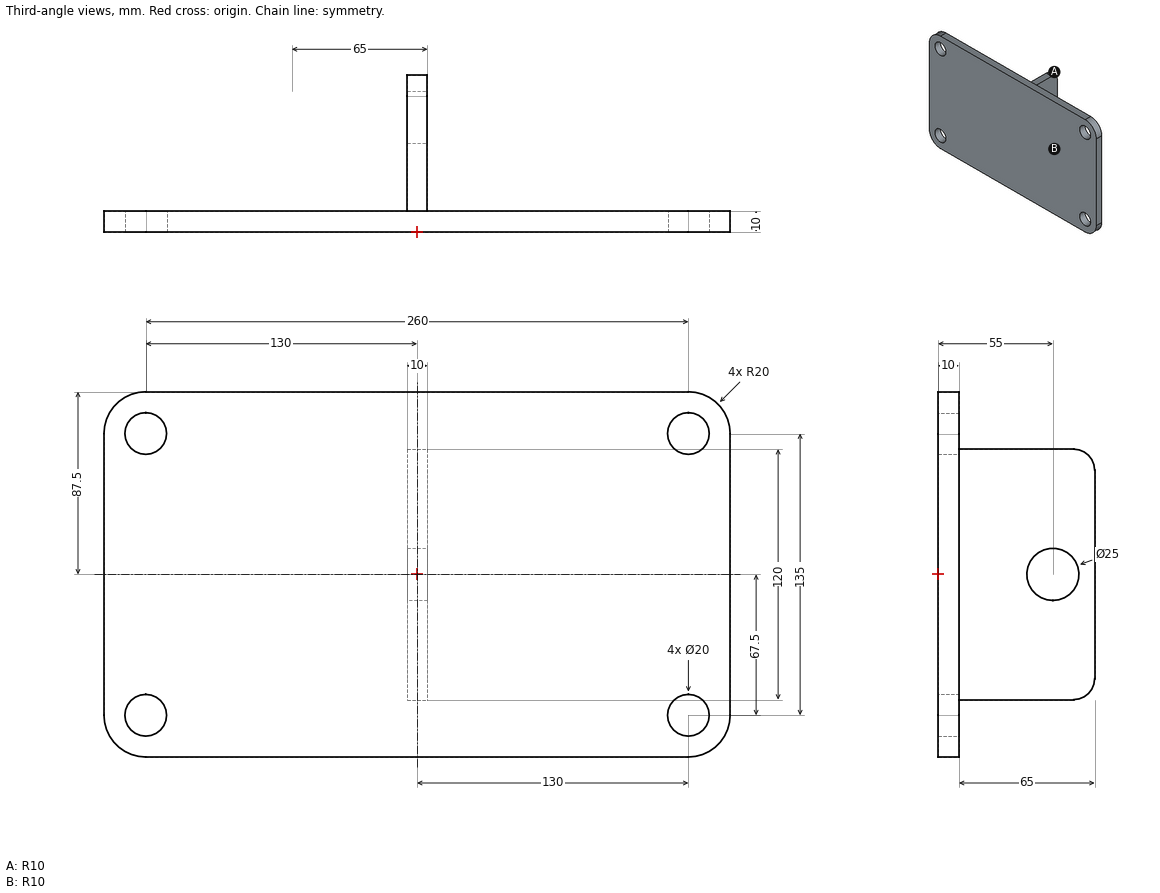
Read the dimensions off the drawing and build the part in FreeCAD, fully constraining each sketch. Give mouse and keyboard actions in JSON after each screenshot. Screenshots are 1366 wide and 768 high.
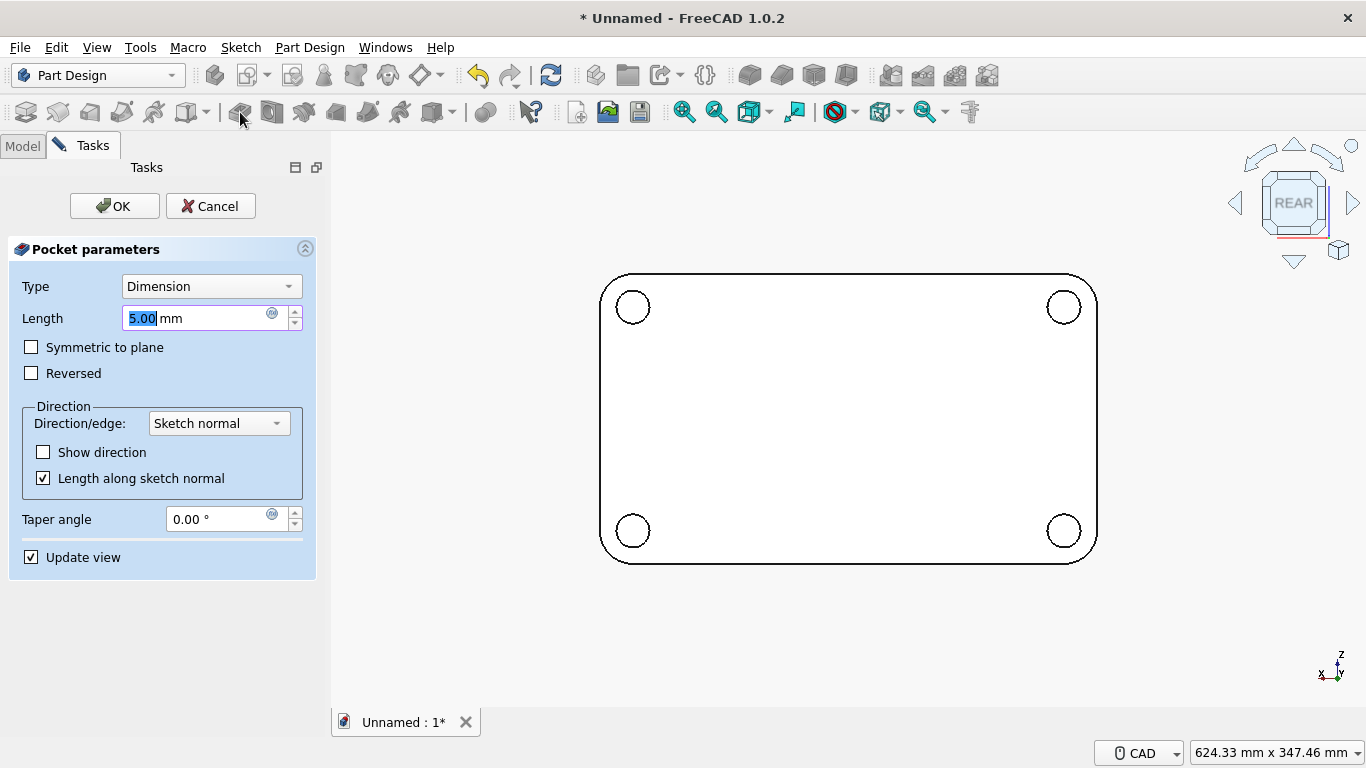
{"action": "type", "text": "10"}
{"action": "key", "text": "Tab"}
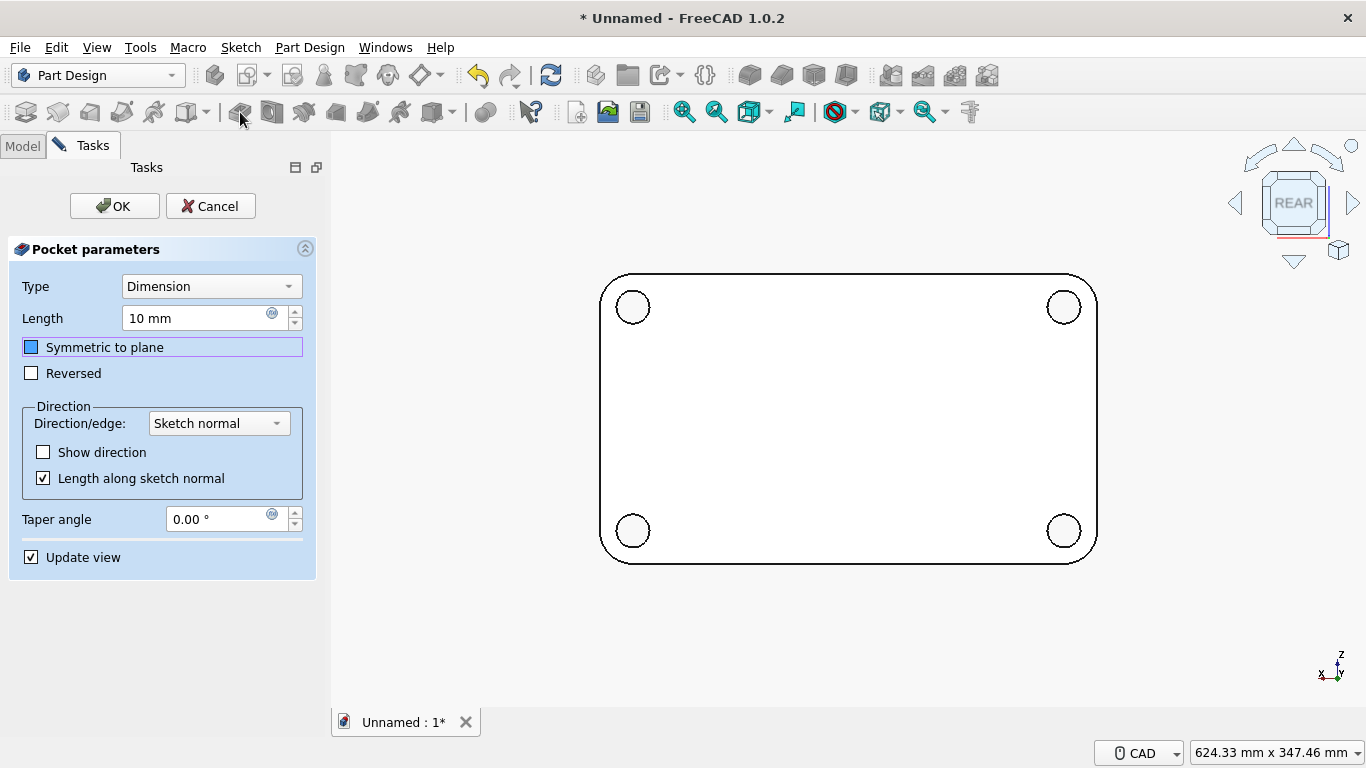
{"action": "left_click", "coordinate": [115, 206]}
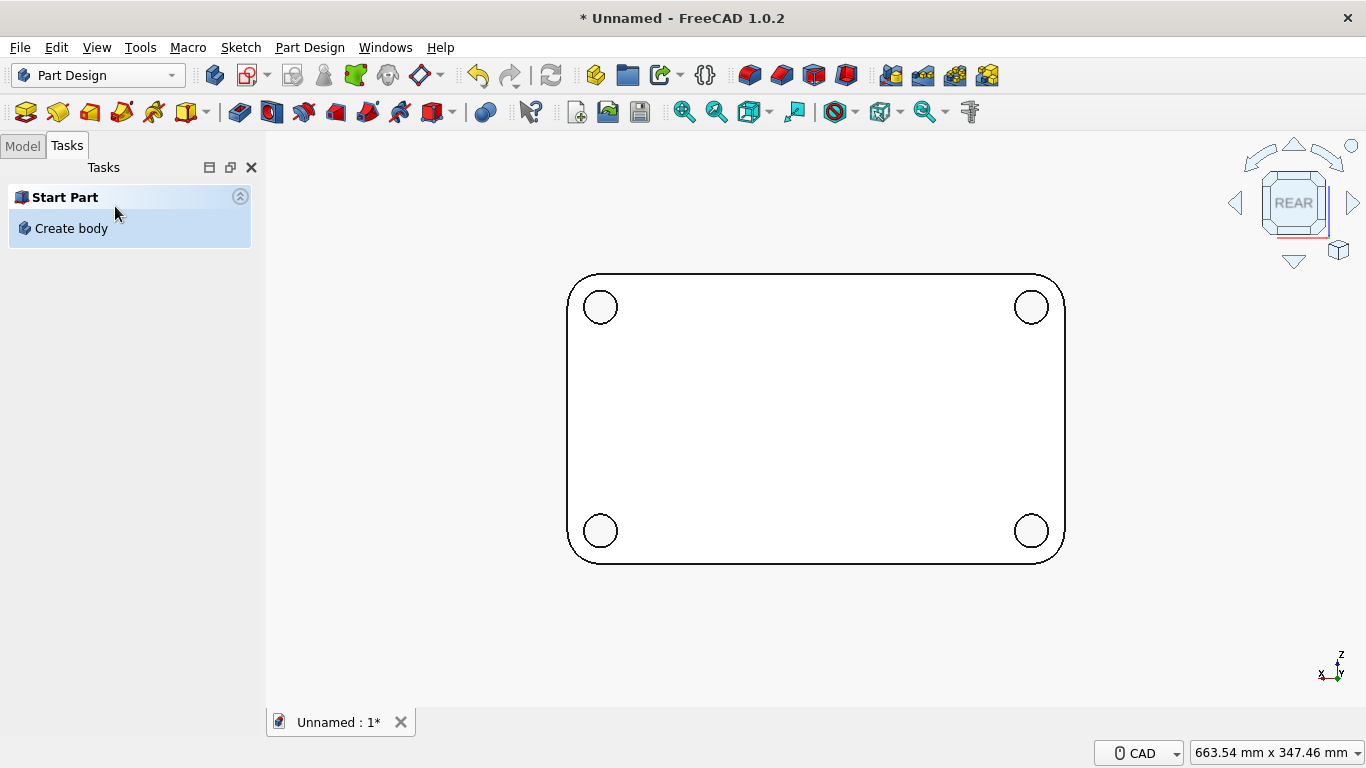
{"action": "left_click", "coordinate": [745, 418]}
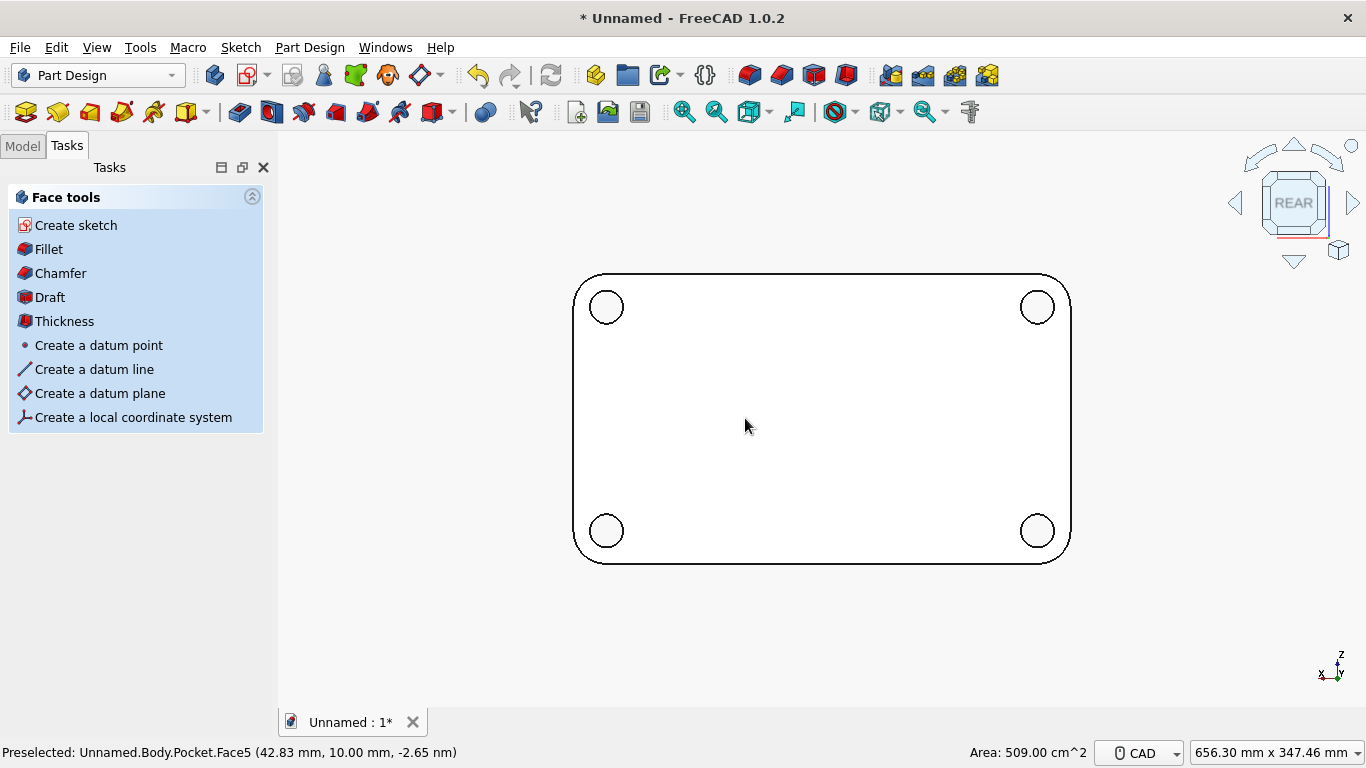
{"action": "left_click", "coordinate": [248, 76]}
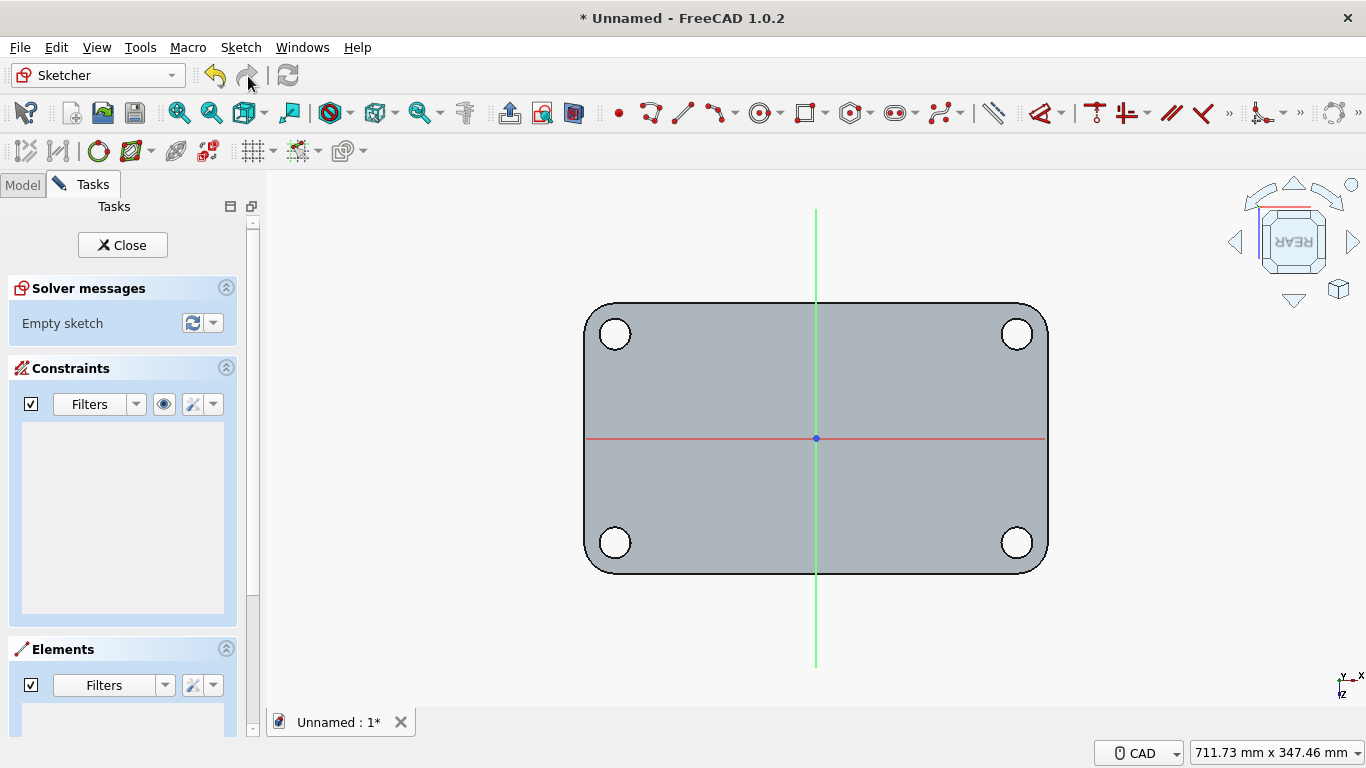
{"action": "scroll", "coordinate": [899, 438], "scroll_direction": "up", "scroll_amount": 3}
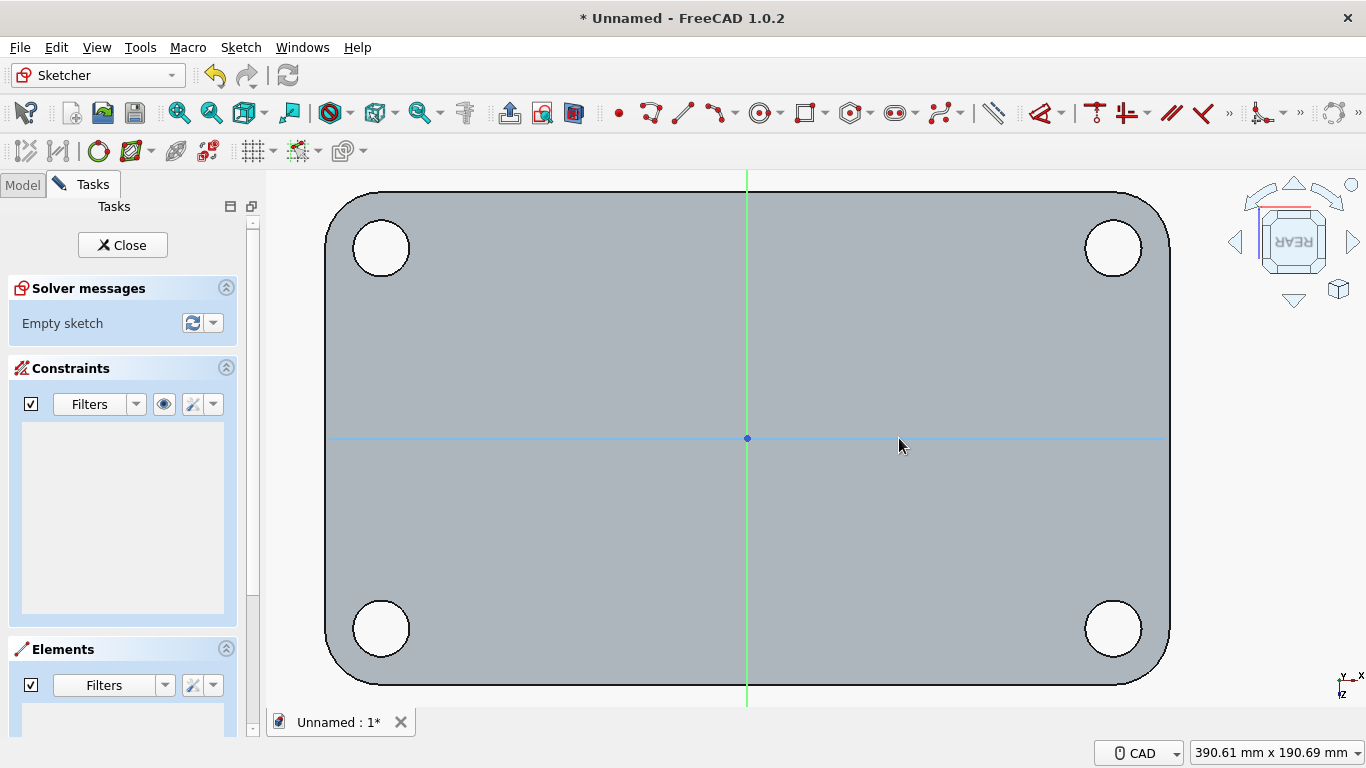
{"action": "key", "text": "g v"}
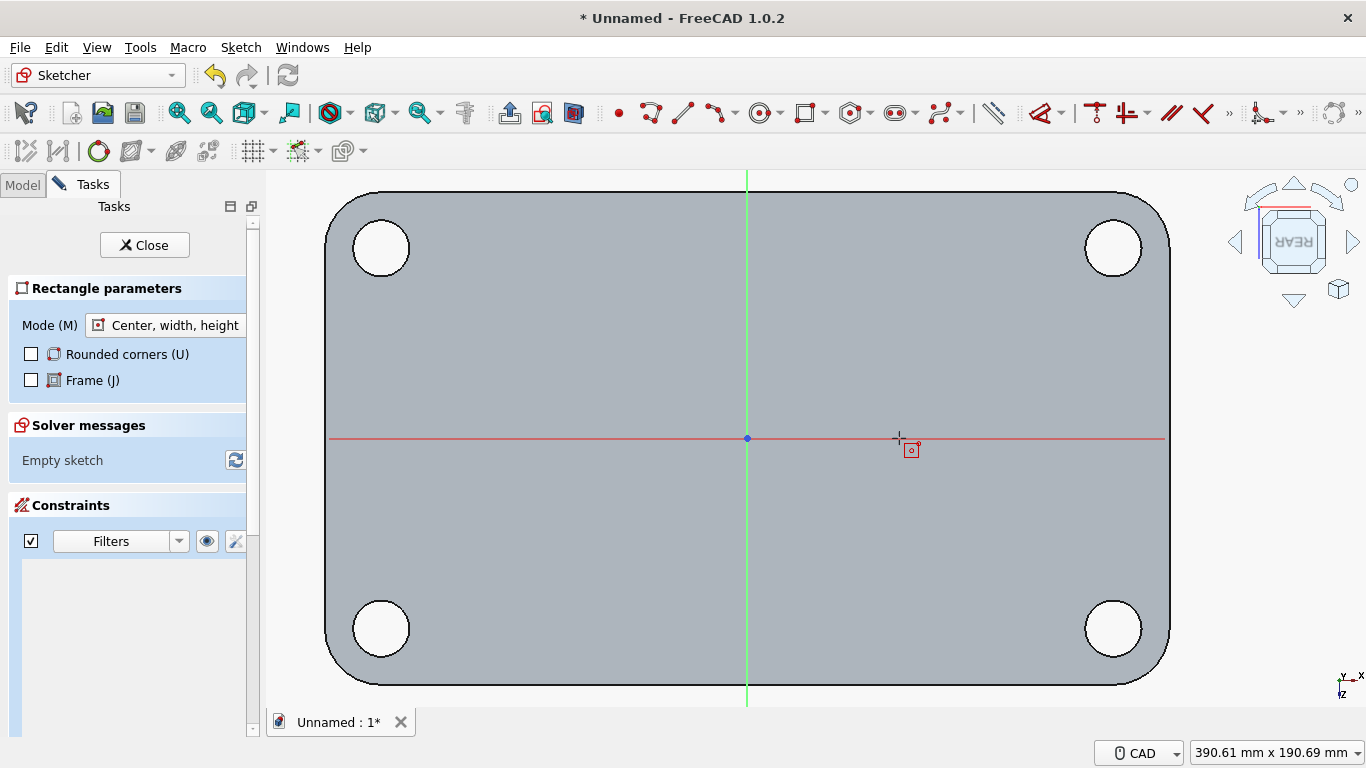
{"action": "left_click", "coordinate": [747, 438]}
{"action": "left_click", "coordinate": [761, 270]}
{"action": "key", "text": "Escape"}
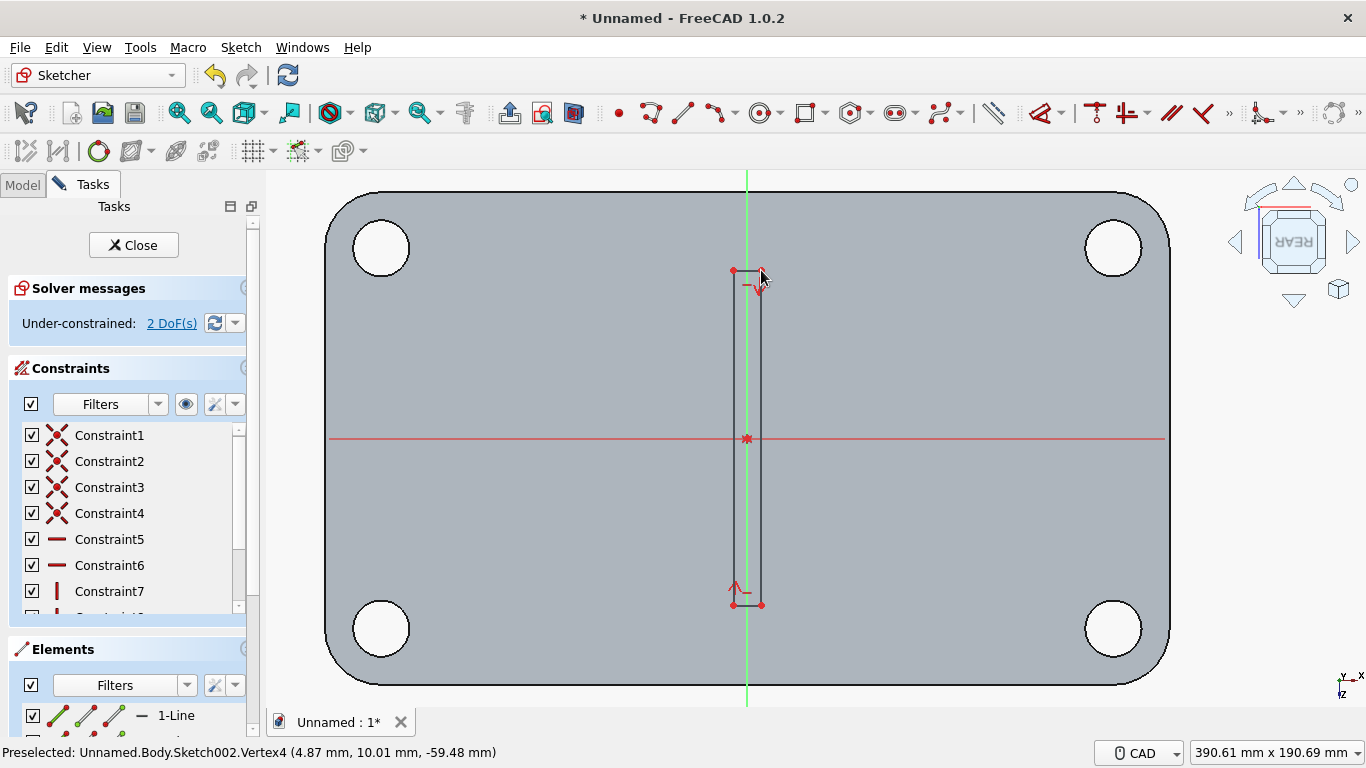
{"action": "left_click", "coordinate": [1040, 114]}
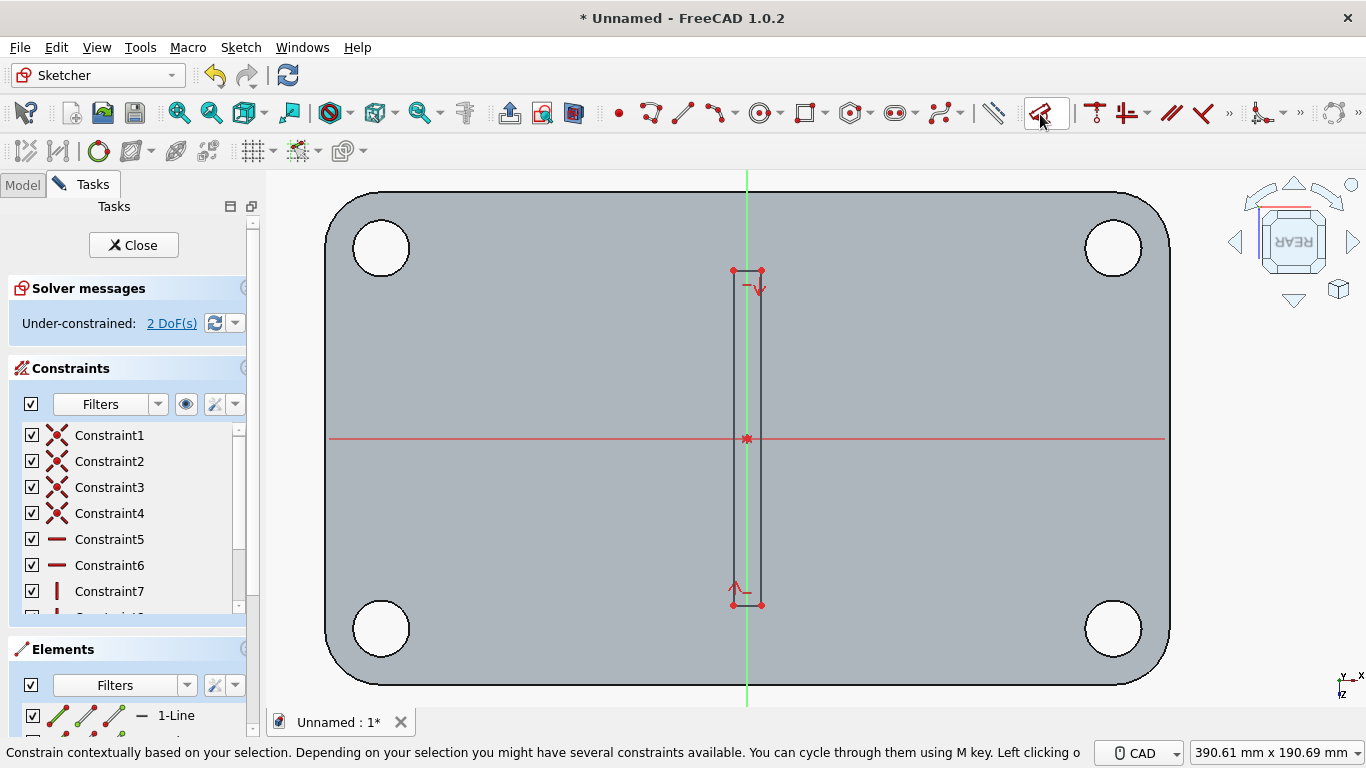
{"action": "scroll", "coordinate": [745, 606], "scroll_direction": "up", "scroll_amount": 2}